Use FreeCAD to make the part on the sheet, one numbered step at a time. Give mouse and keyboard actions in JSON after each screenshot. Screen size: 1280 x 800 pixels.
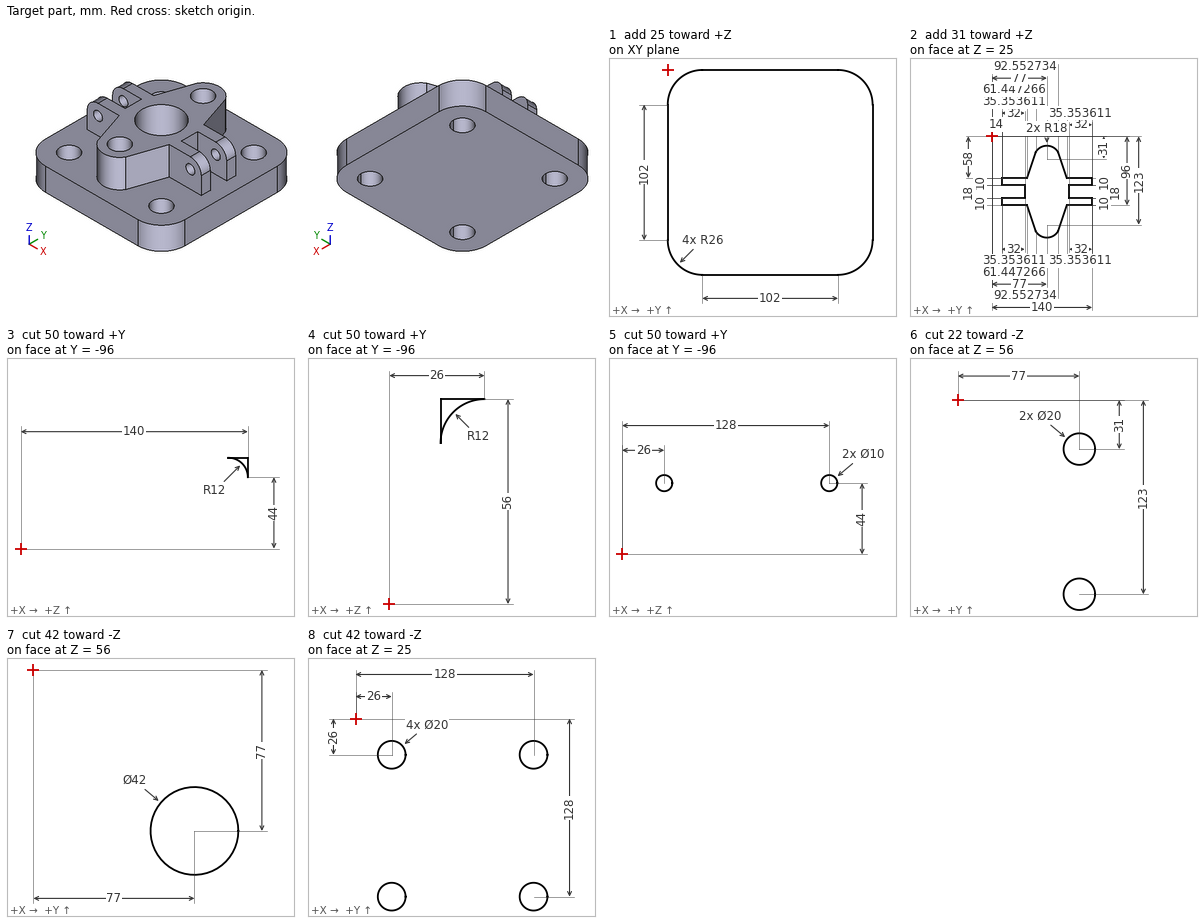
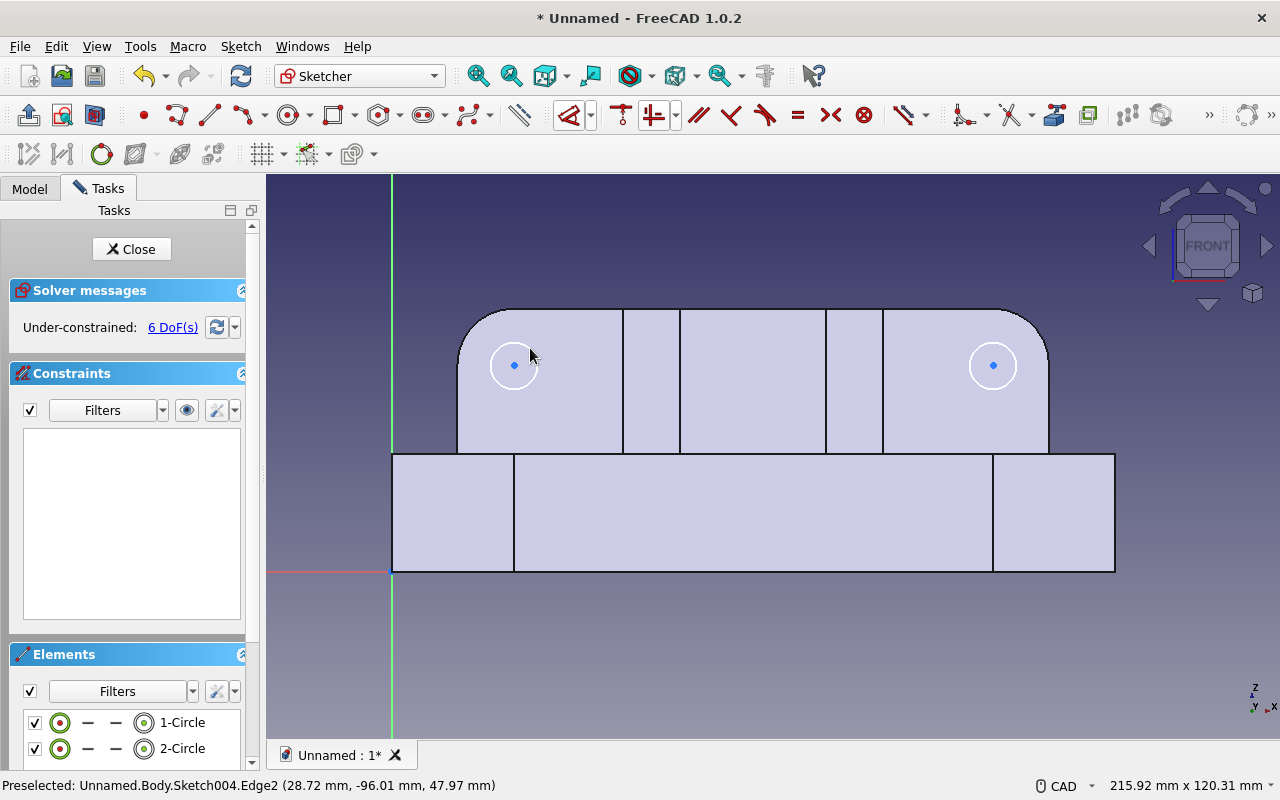
{"action": "left_click", "coordinate": [1009, 349]}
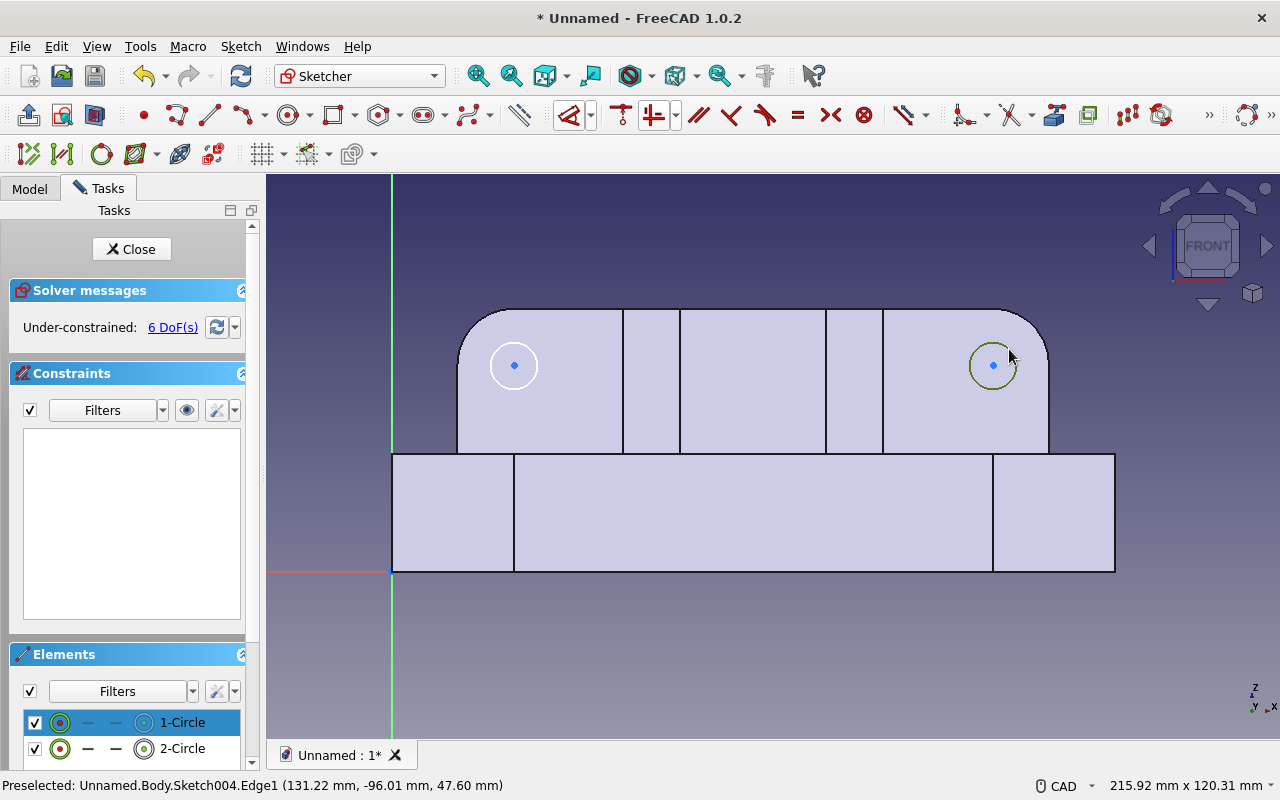
{"action": "left_click", "coordinate": [530, 349]}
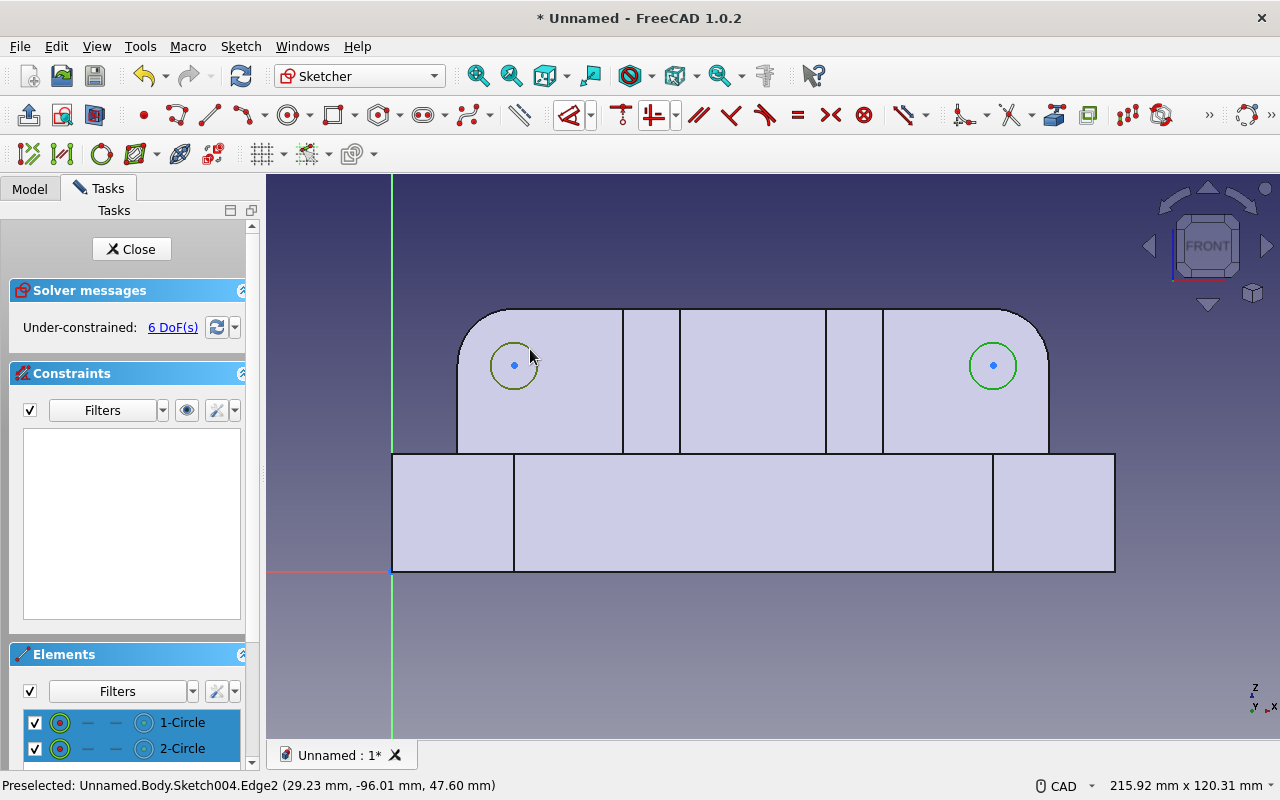
{"action": "left_click", "coordinate": [798, 116]}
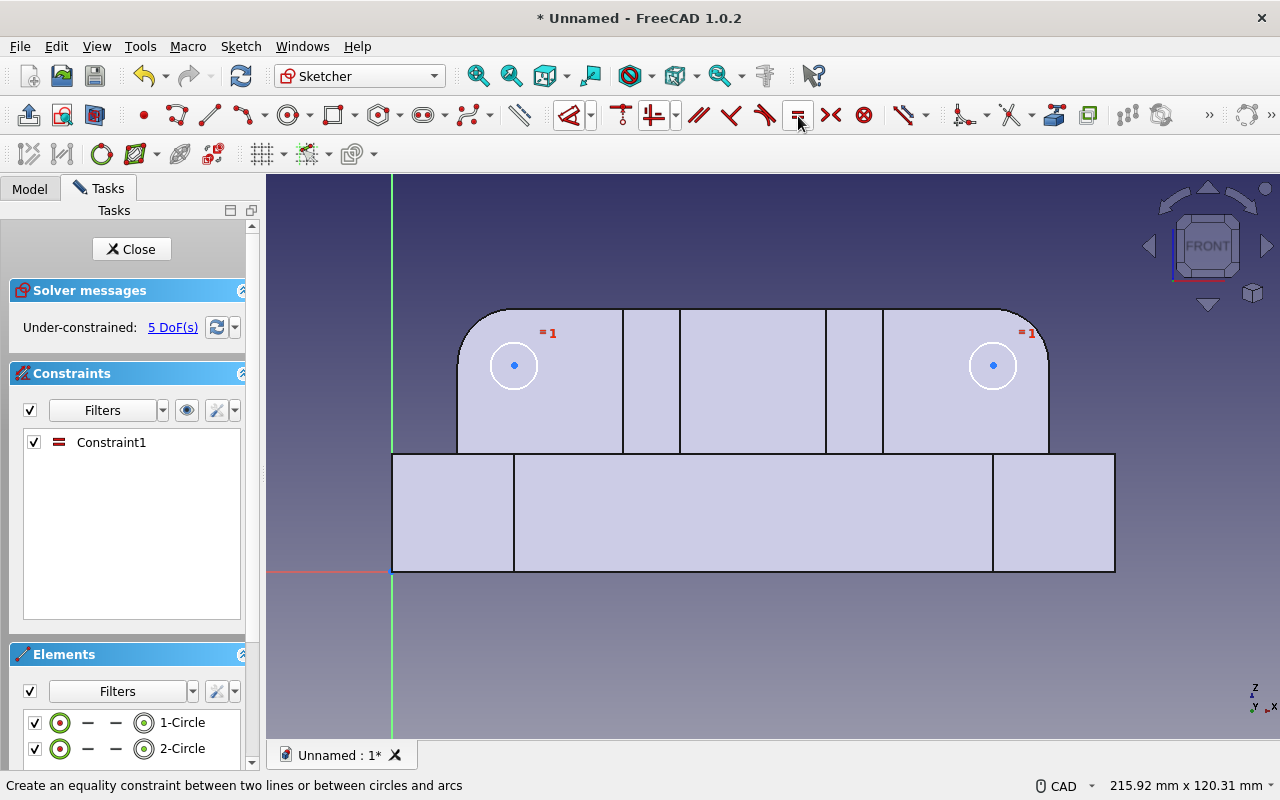
{"action": "left_click", "coordinate": [993, 366]}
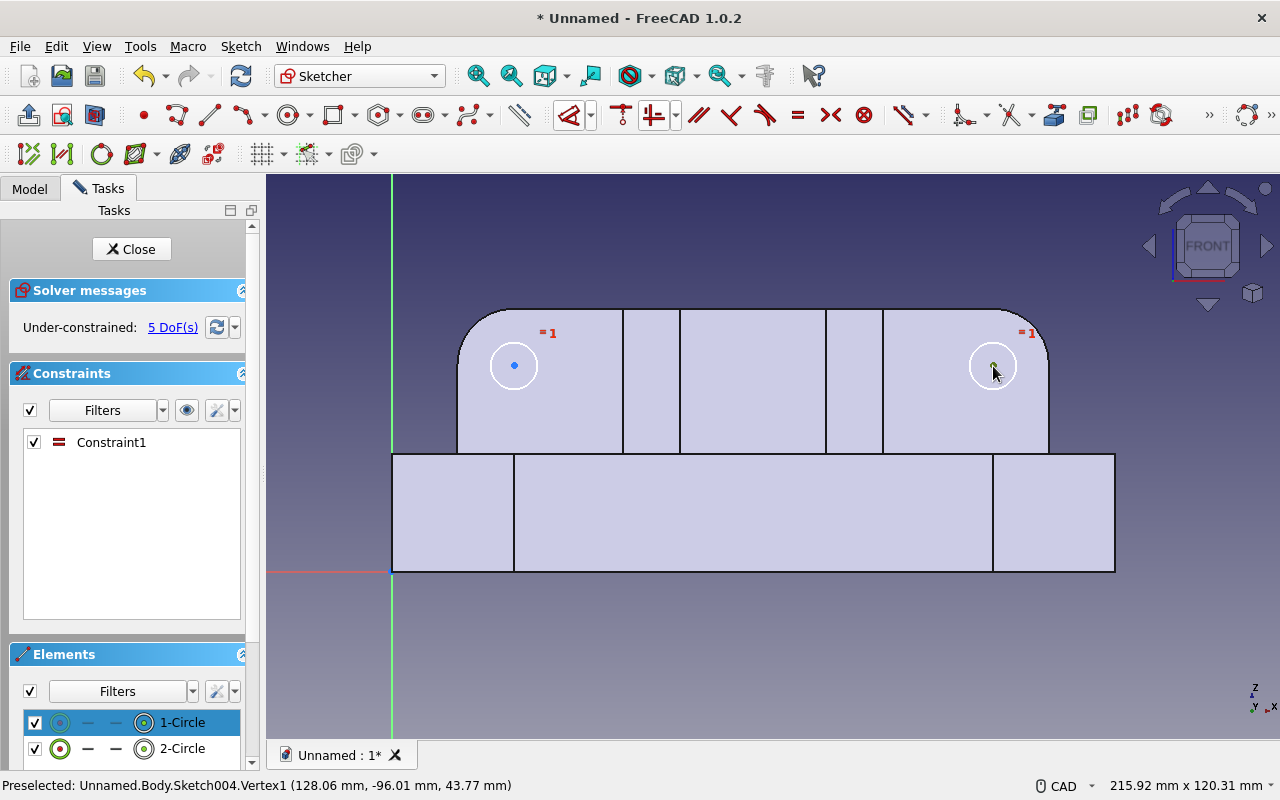
{"action": "left_click", "coordinate": [514, 366]}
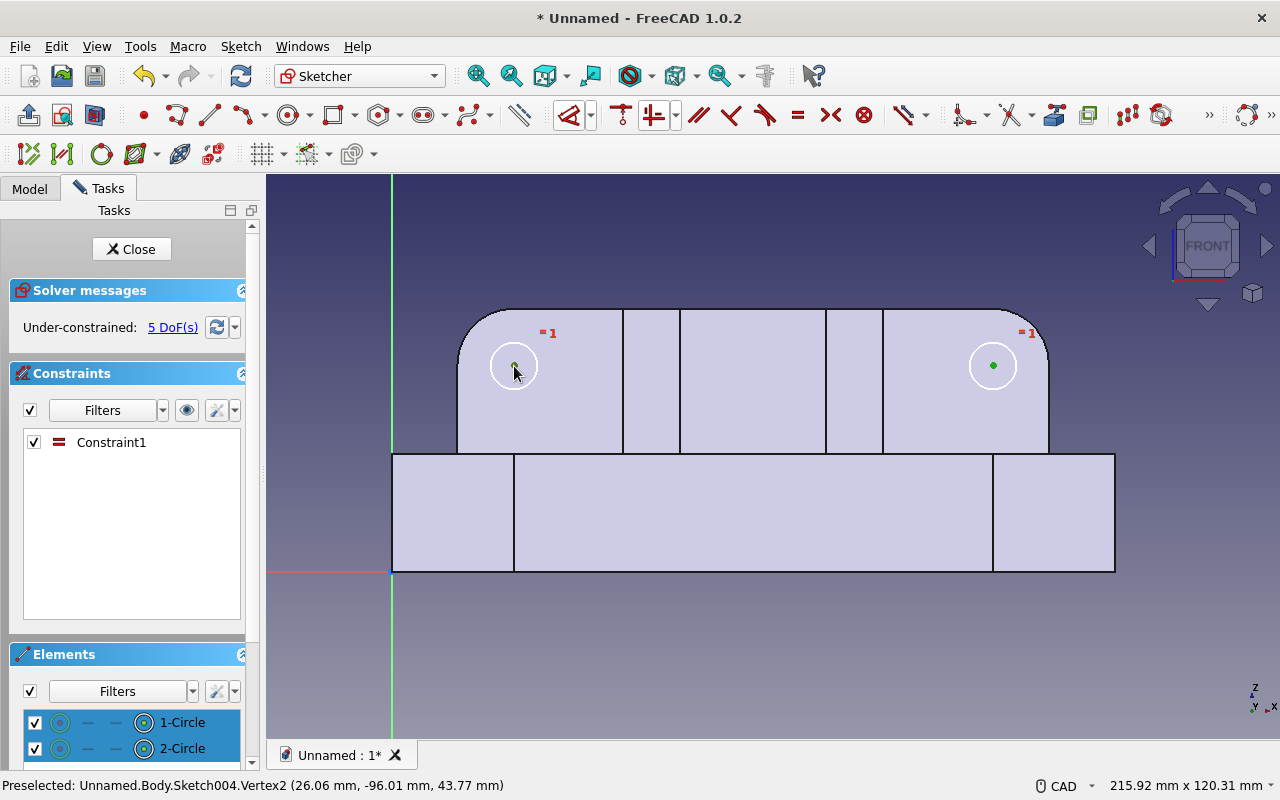
{"action": "key", "text": "h"}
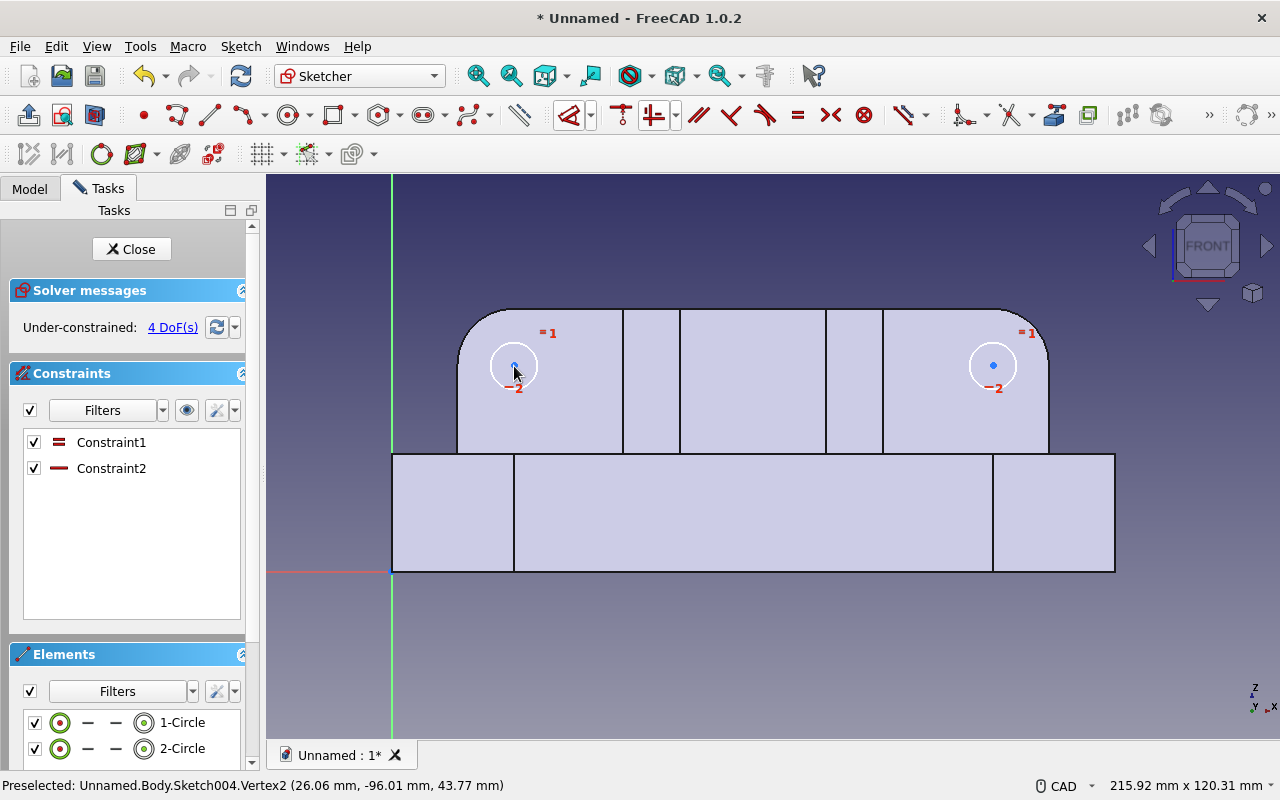
{"action": "left_click", "coordinate": [1009, 349]}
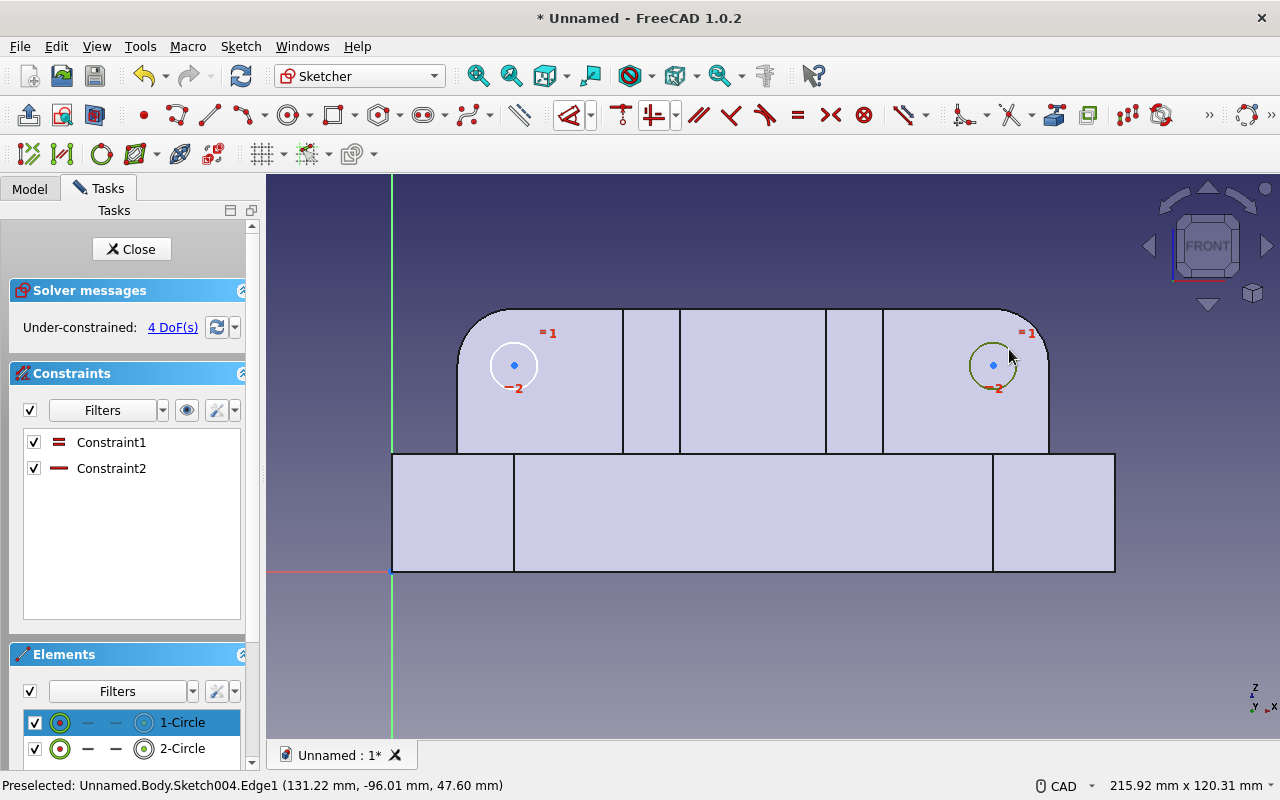
{"action": "left_click", "coordinate": [590, 116]}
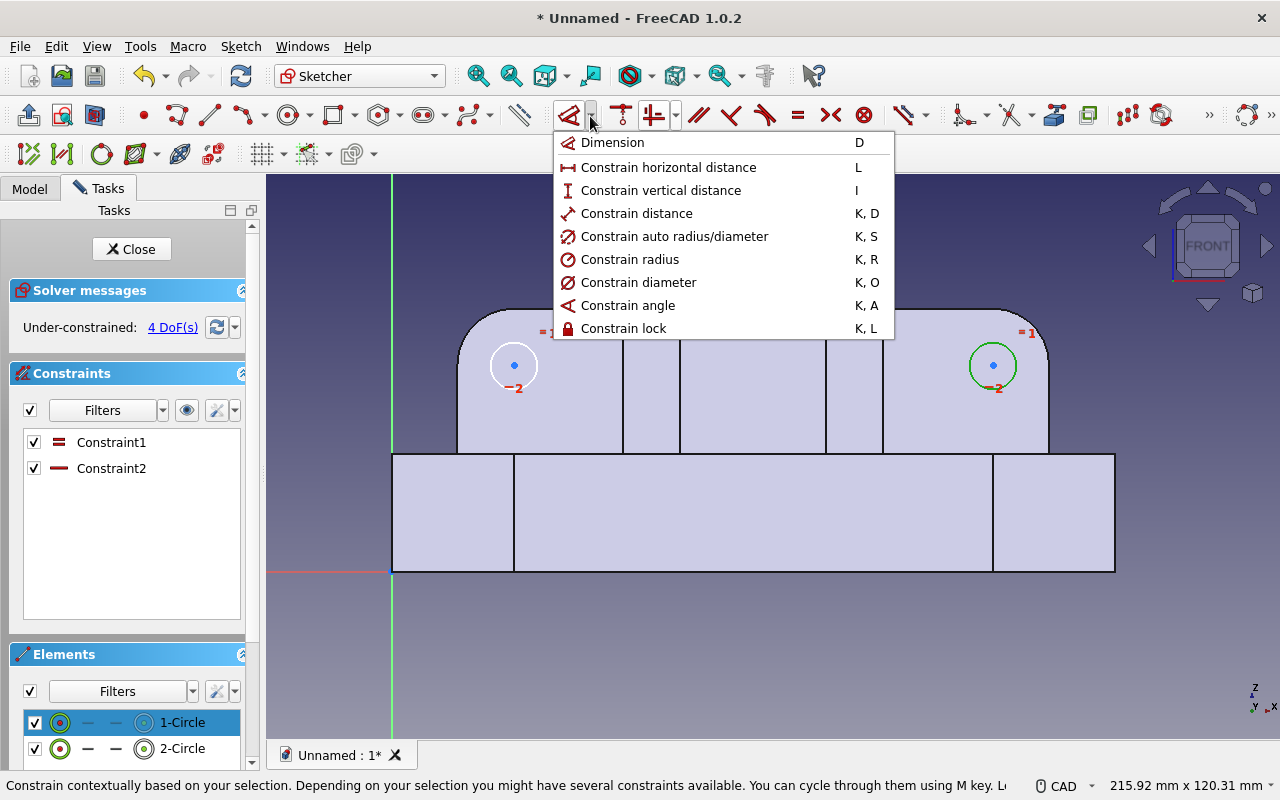
{"action": "left_click", "coordinate": [724, 282]}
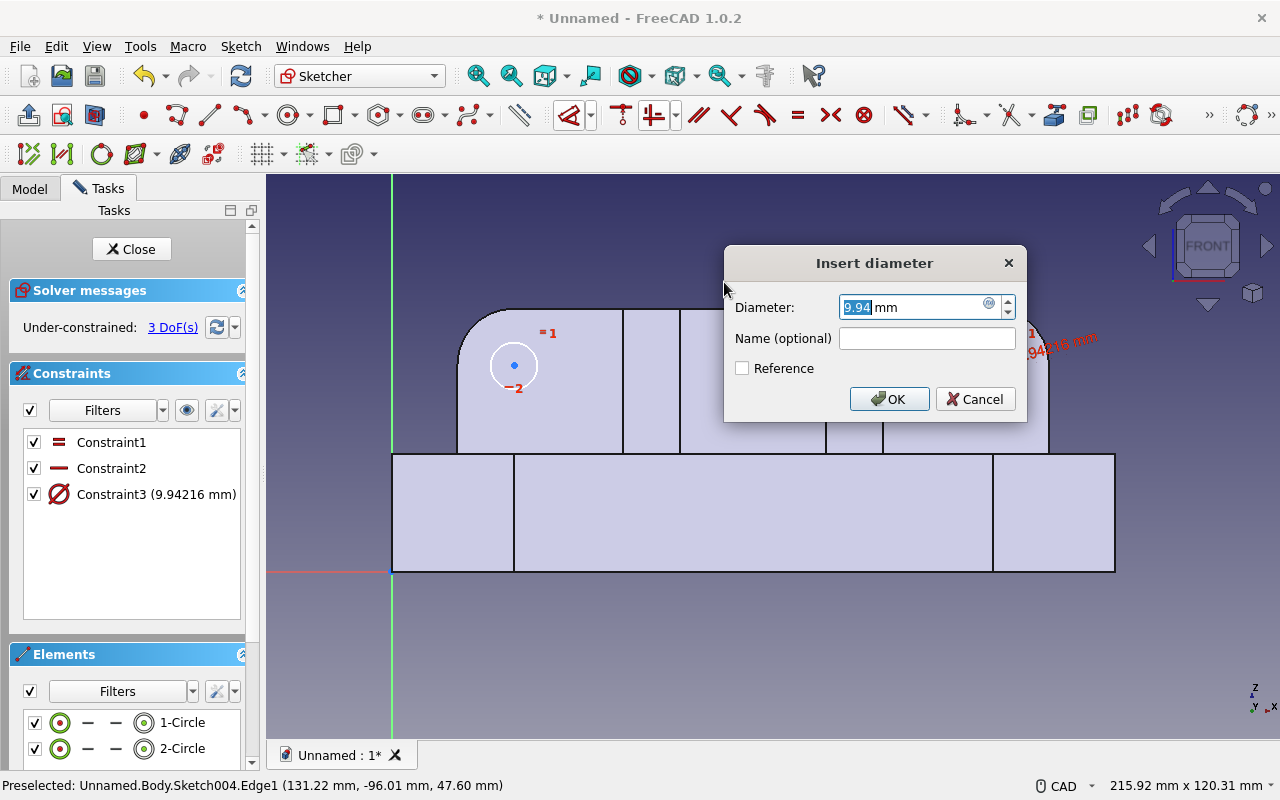
{"action": "type", "text": "10"}
{"action": "key", "text": "Return"}